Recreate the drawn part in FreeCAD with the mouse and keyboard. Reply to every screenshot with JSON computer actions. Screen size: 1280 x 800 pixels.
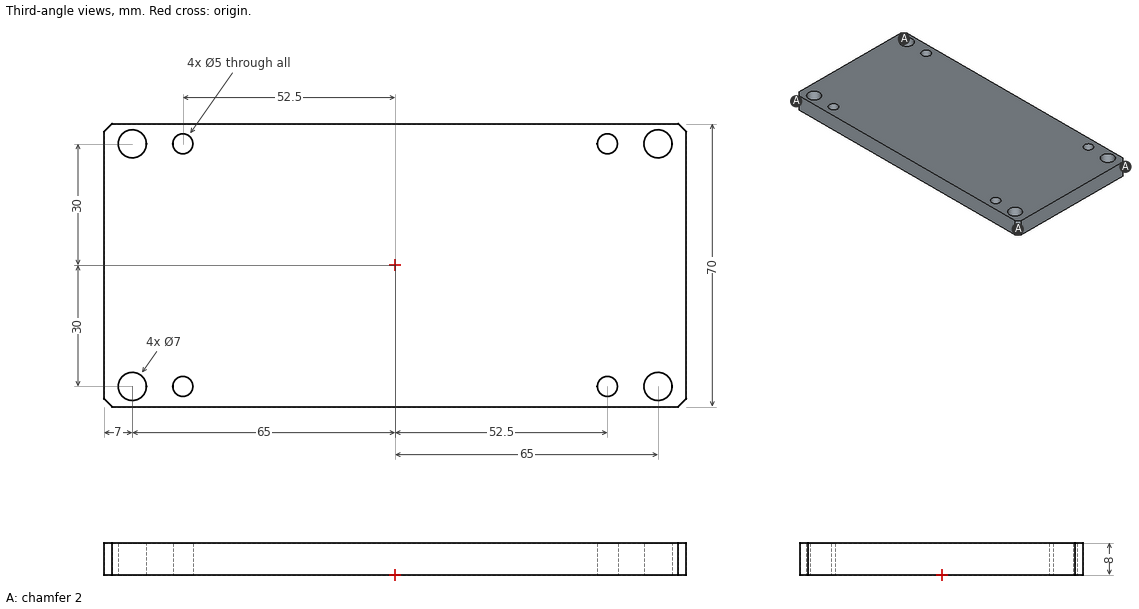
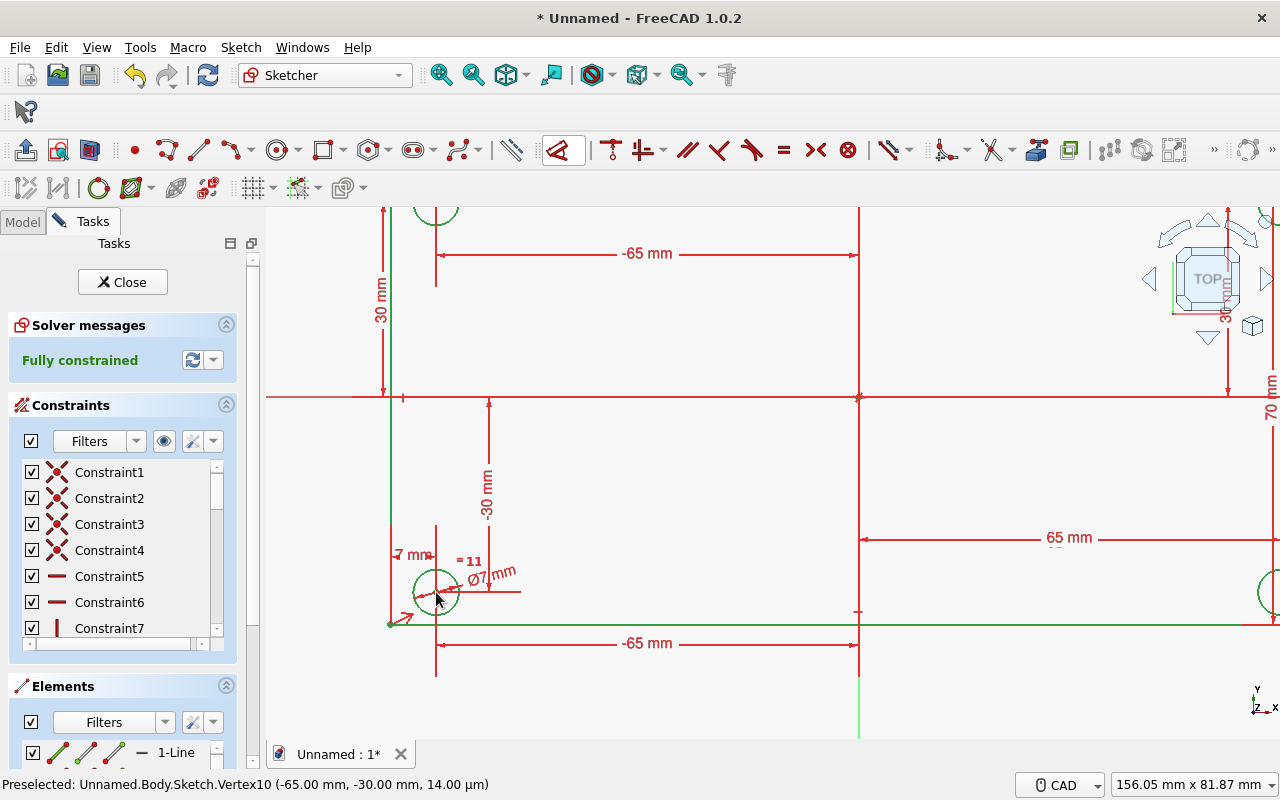
{"action": "left_click", "coordinate": [123, 282]}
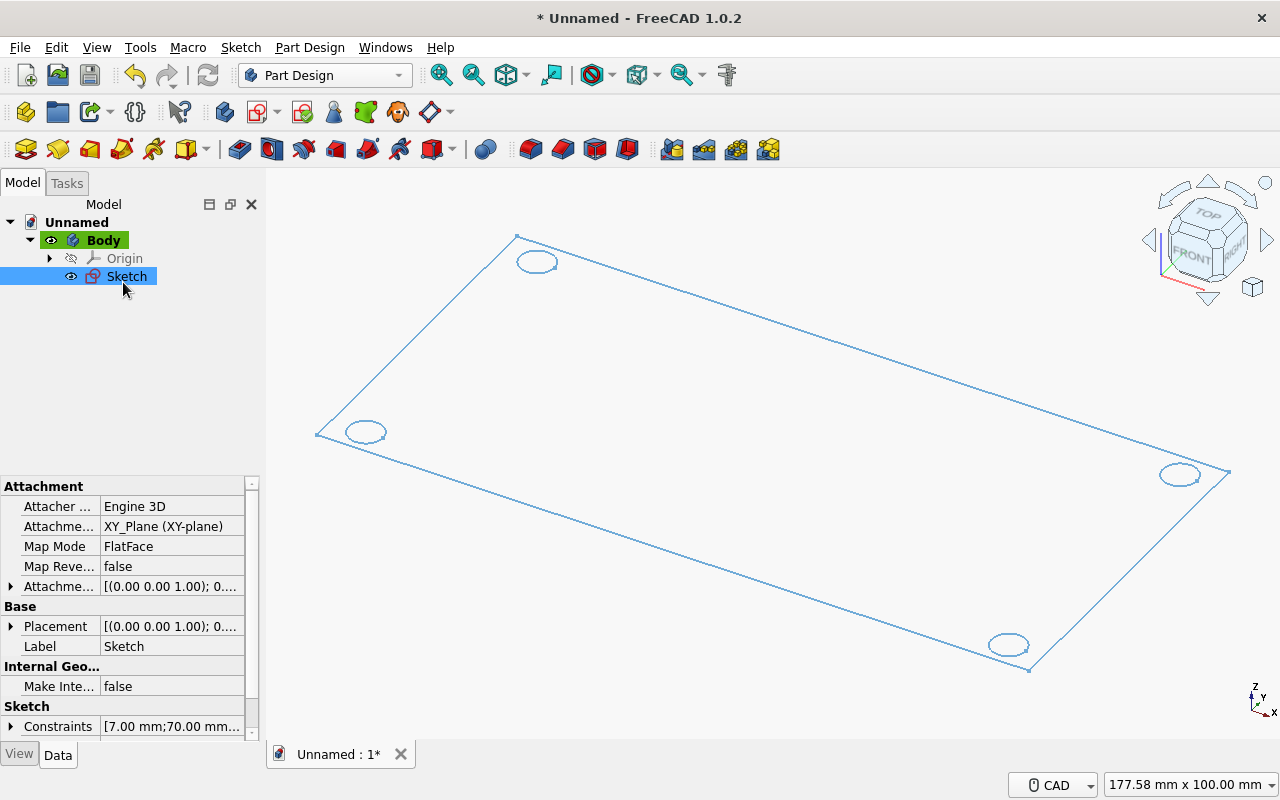
{"action": "left_click", "coordinate": [26, 150]}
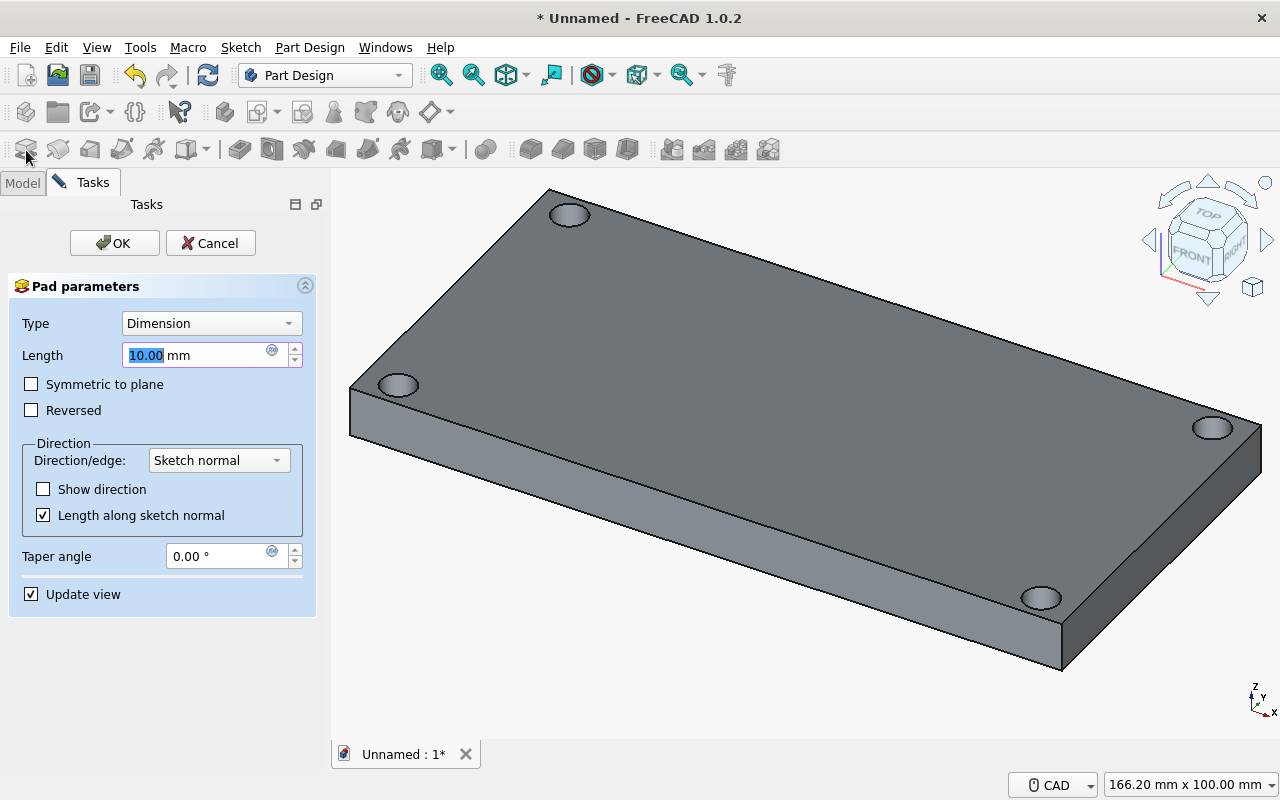
{"action": "type", "text": "8"}
{"action": "key", "text": "Tab"}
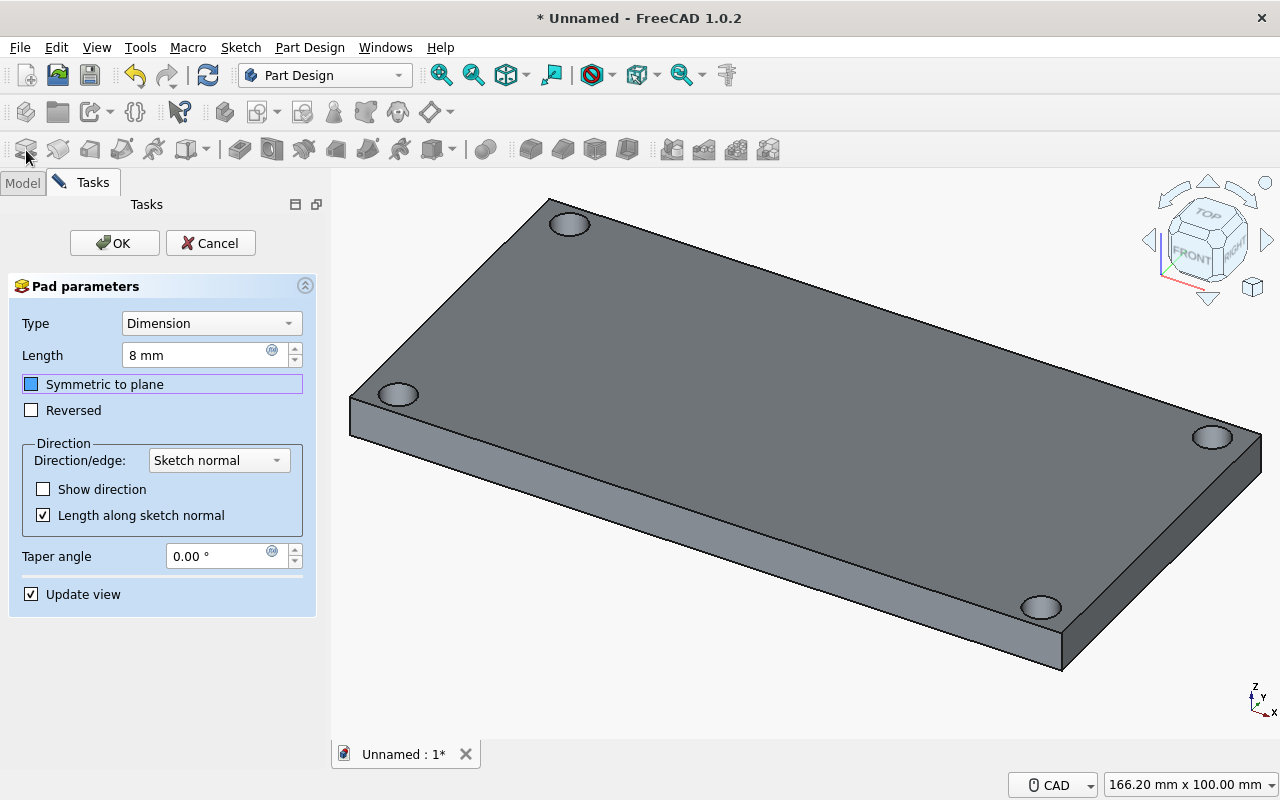
{"action": "left_click", "coordinate": [115, 243]}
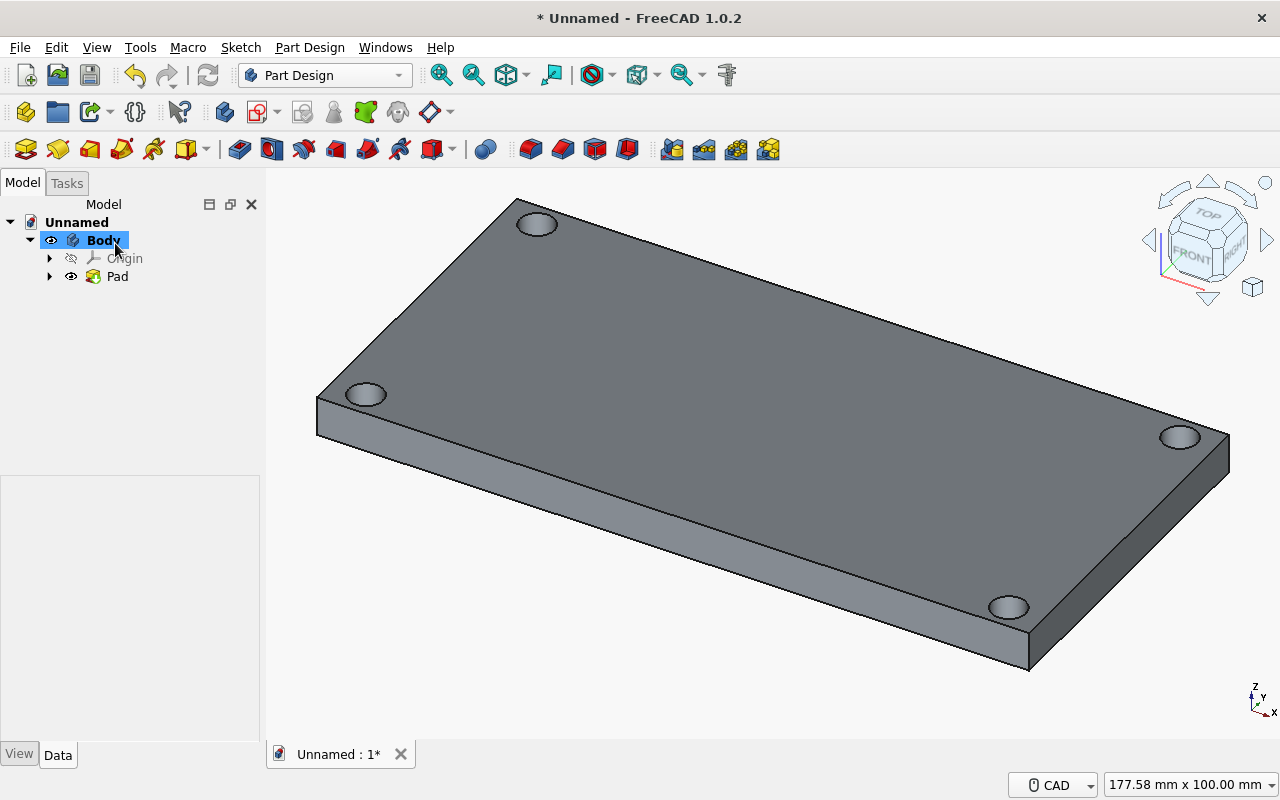
{"action": "left_click", "coordinate": [1029, 651]}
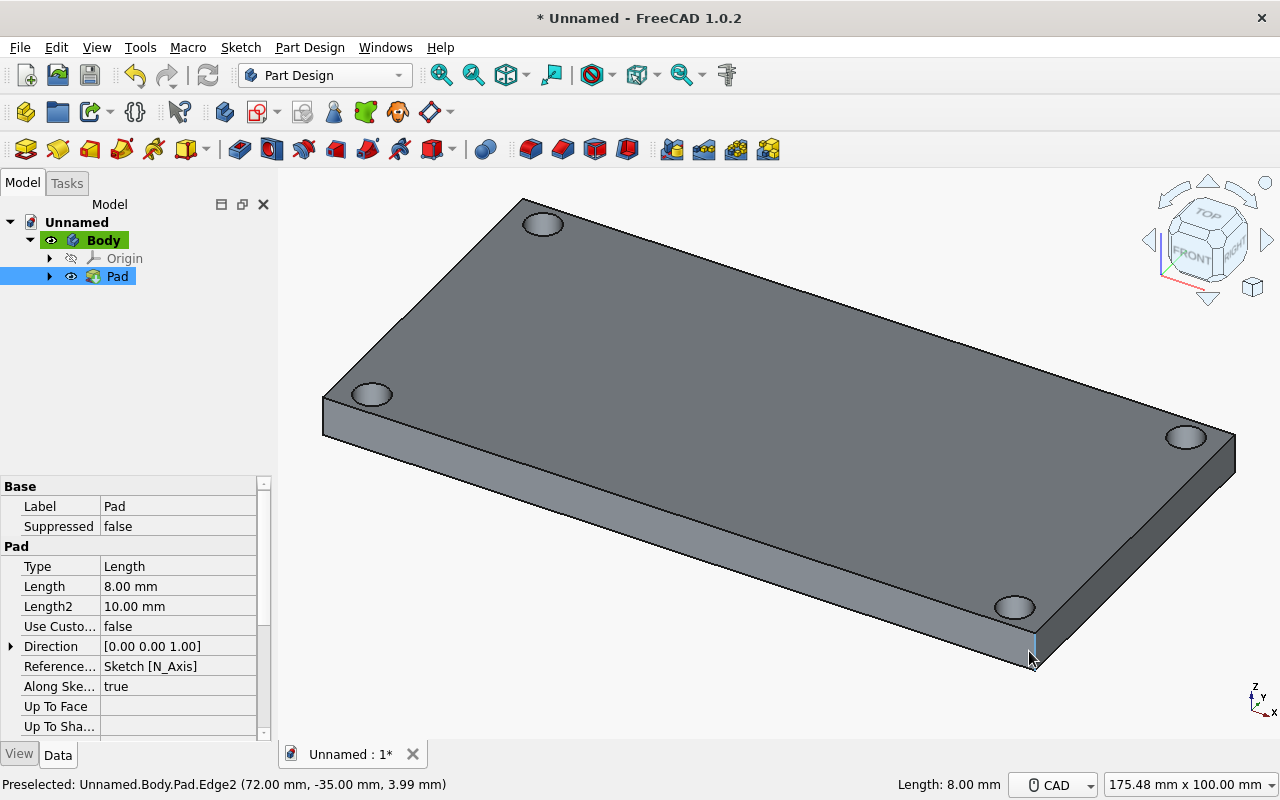
{"action": "key", "text": "0"}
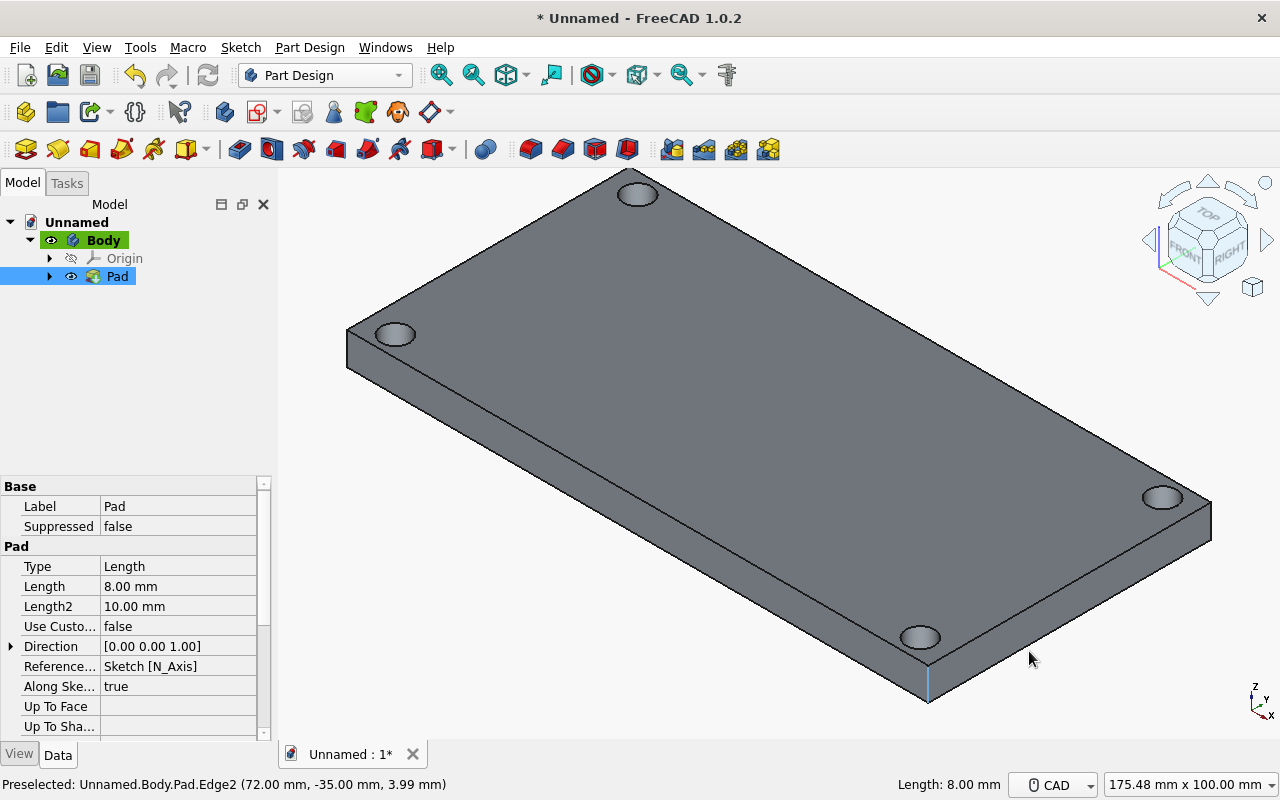
{"action": "key", "text": "v f"}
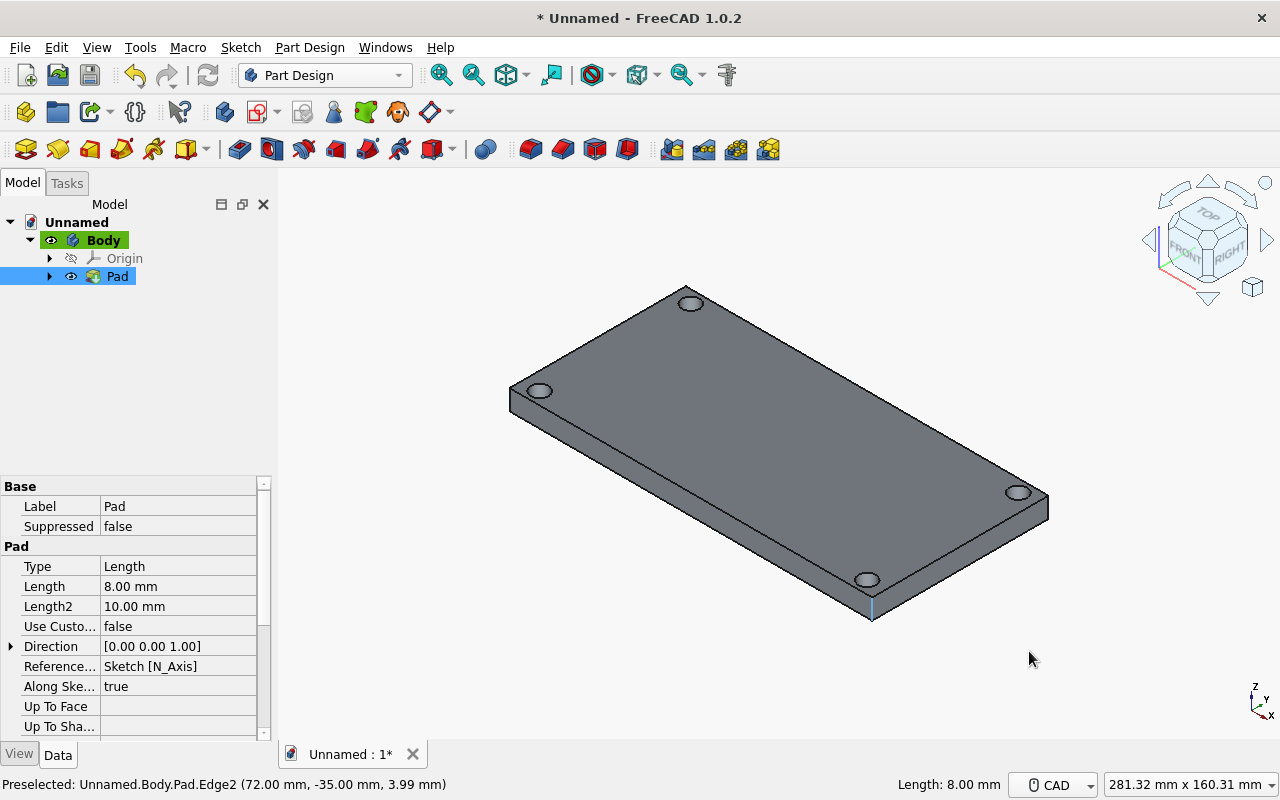
{"action": "key", "text": "2"}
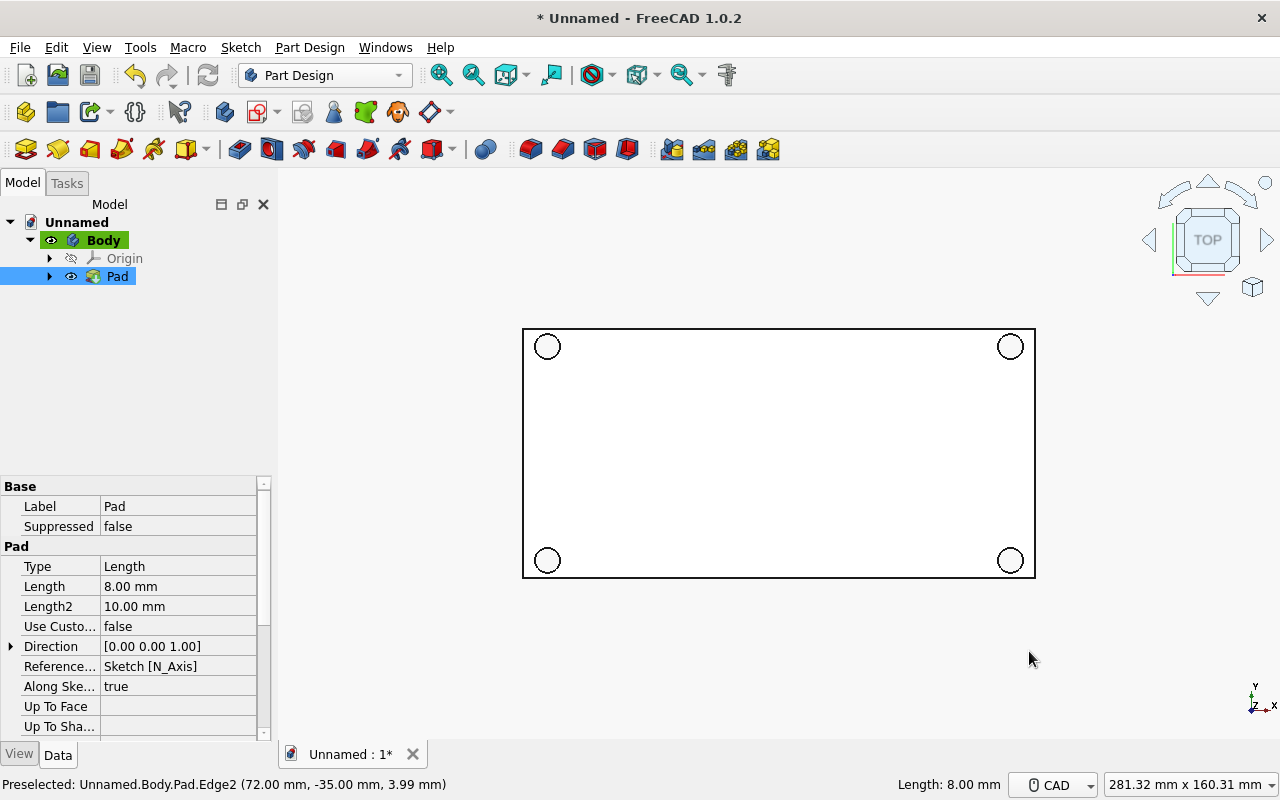
{"action": "key", "text": "1"}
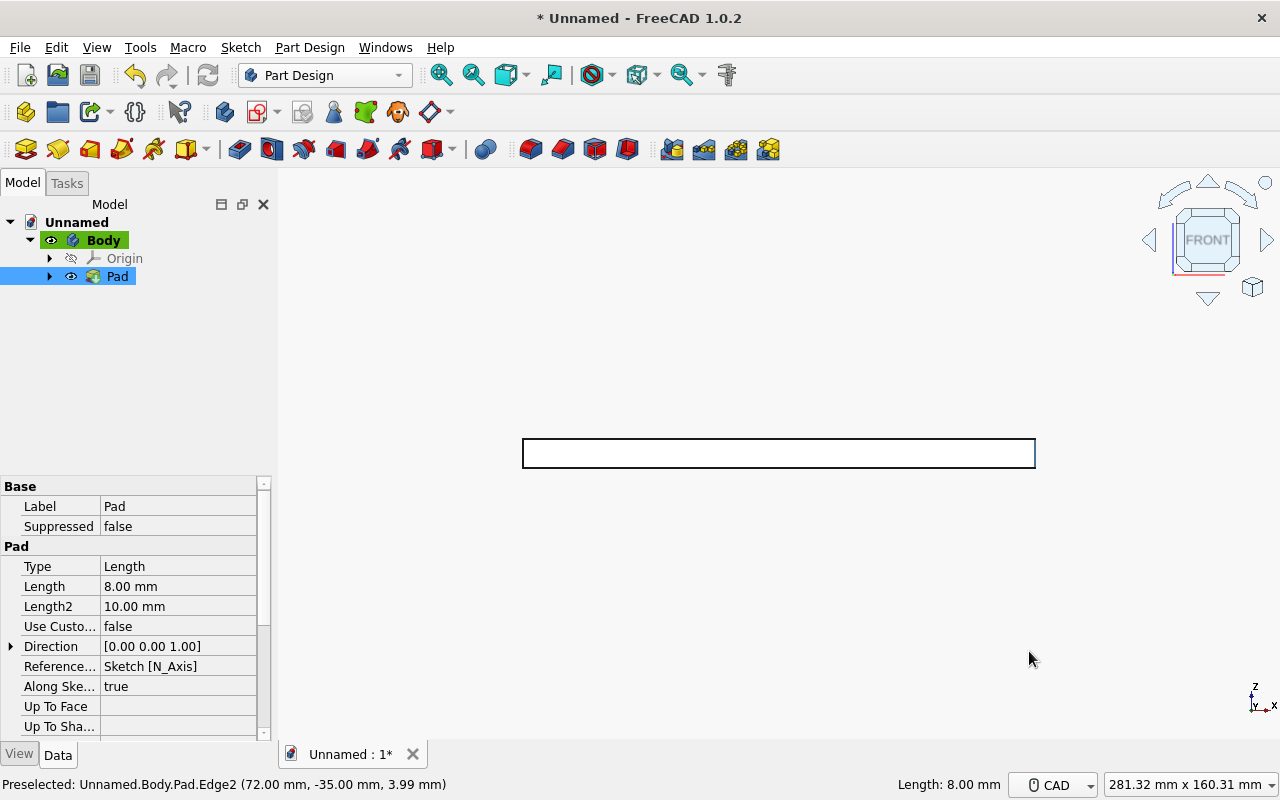
{"action": "left_click", "coordinate": [523, 452], "text": "ctrl"}